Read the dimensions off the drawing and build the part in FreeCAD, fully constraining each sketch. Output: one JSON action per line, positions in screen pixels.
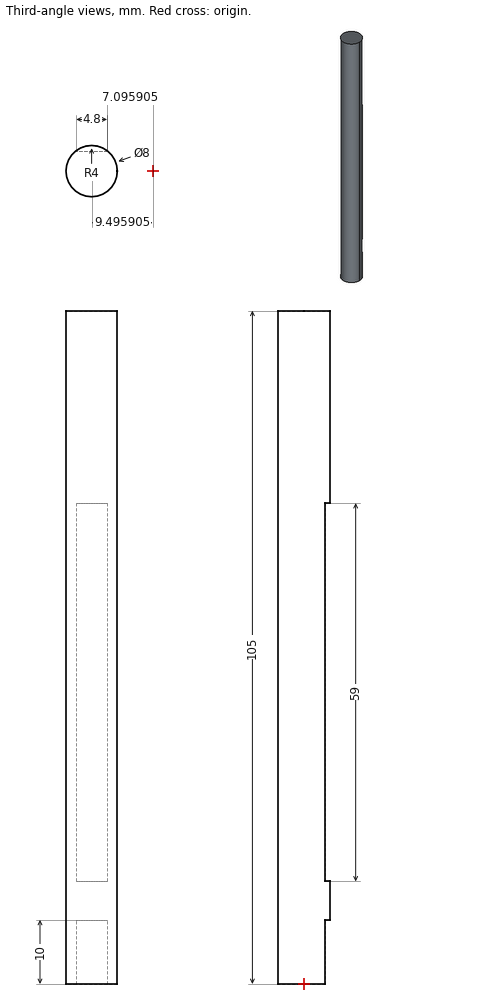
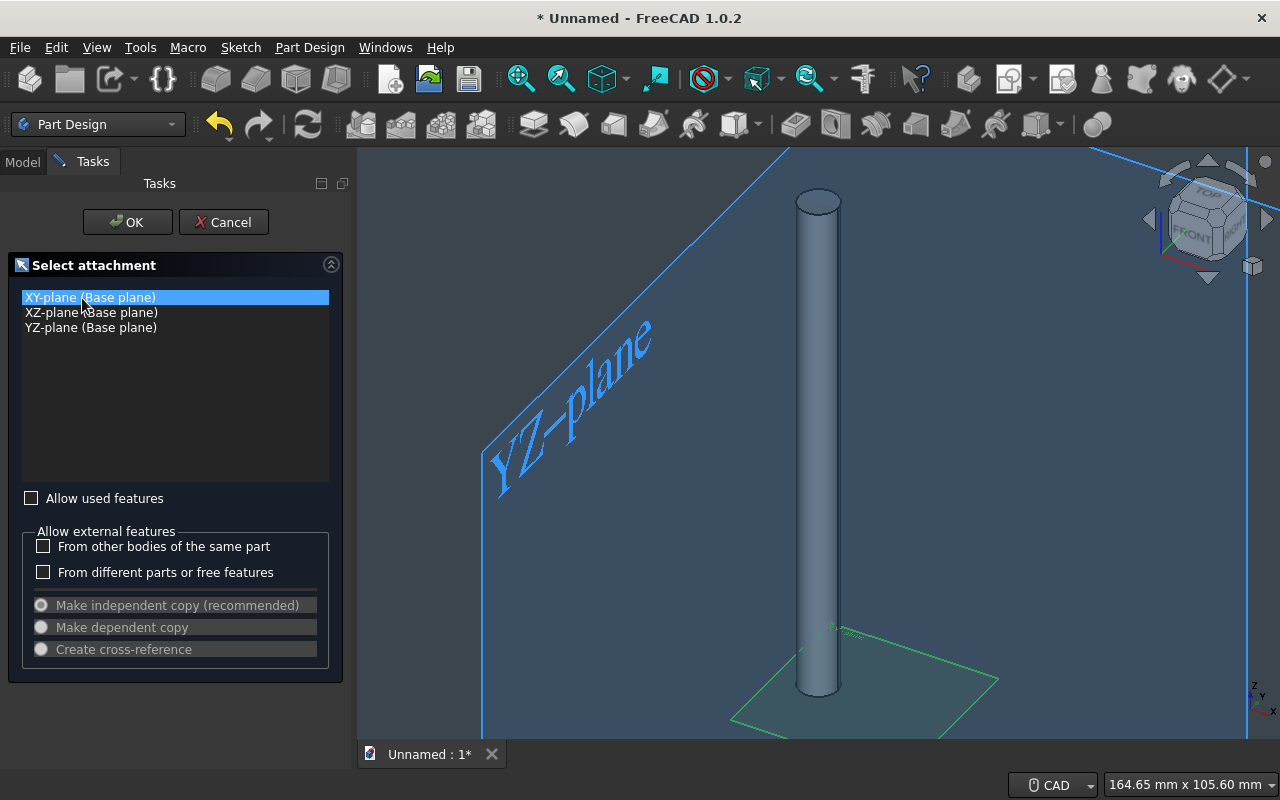
{"action": "left_click", "coordinate": [128, 222]}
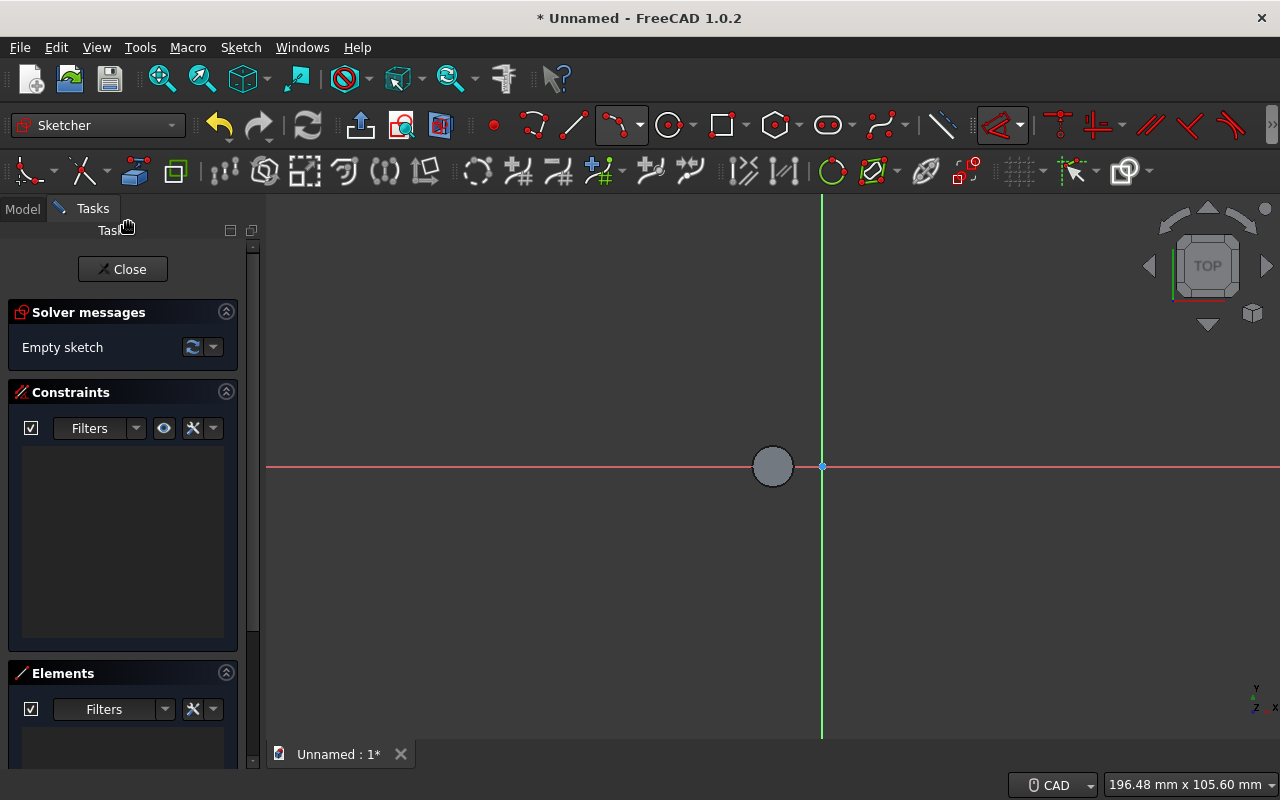
{"action": "key", "text": "q s"}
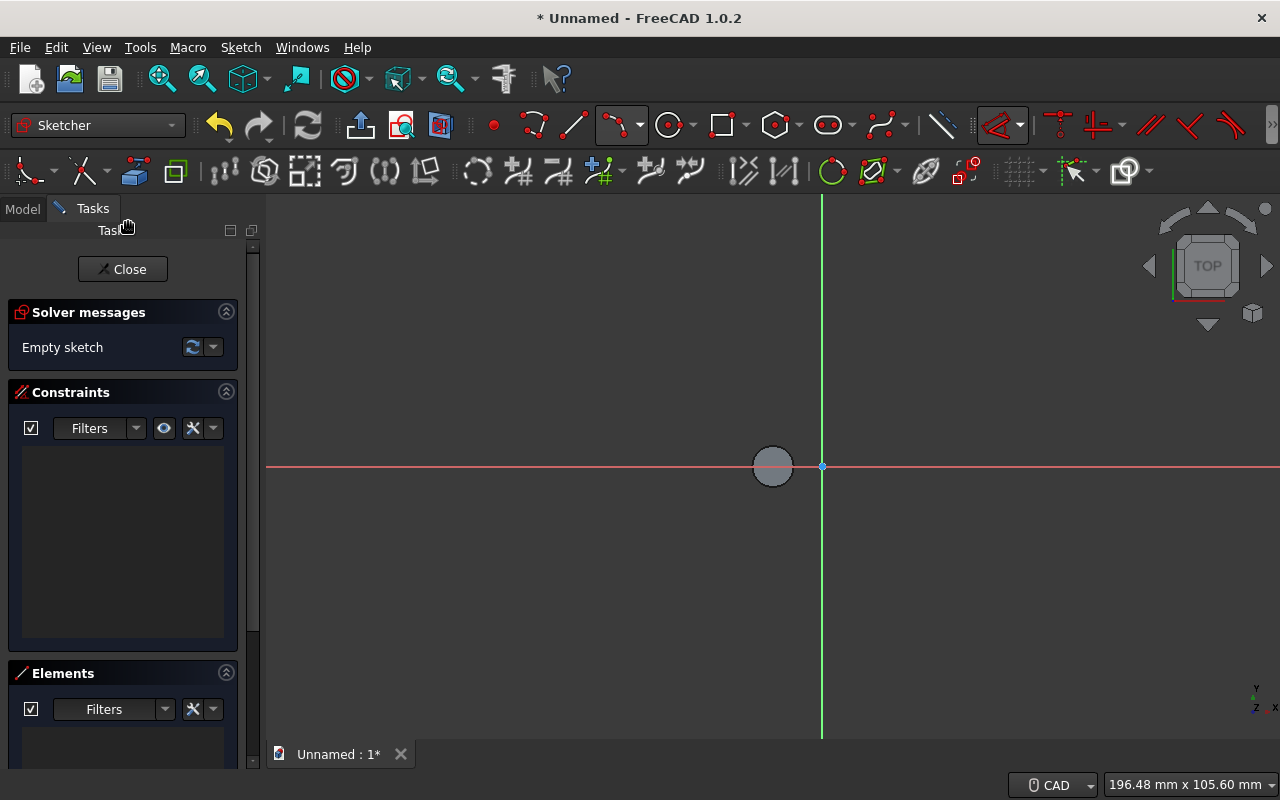
{"action": "scroll", "coordinate": [802, 455], "scroll_direction": "up", "scroll_amount": 11}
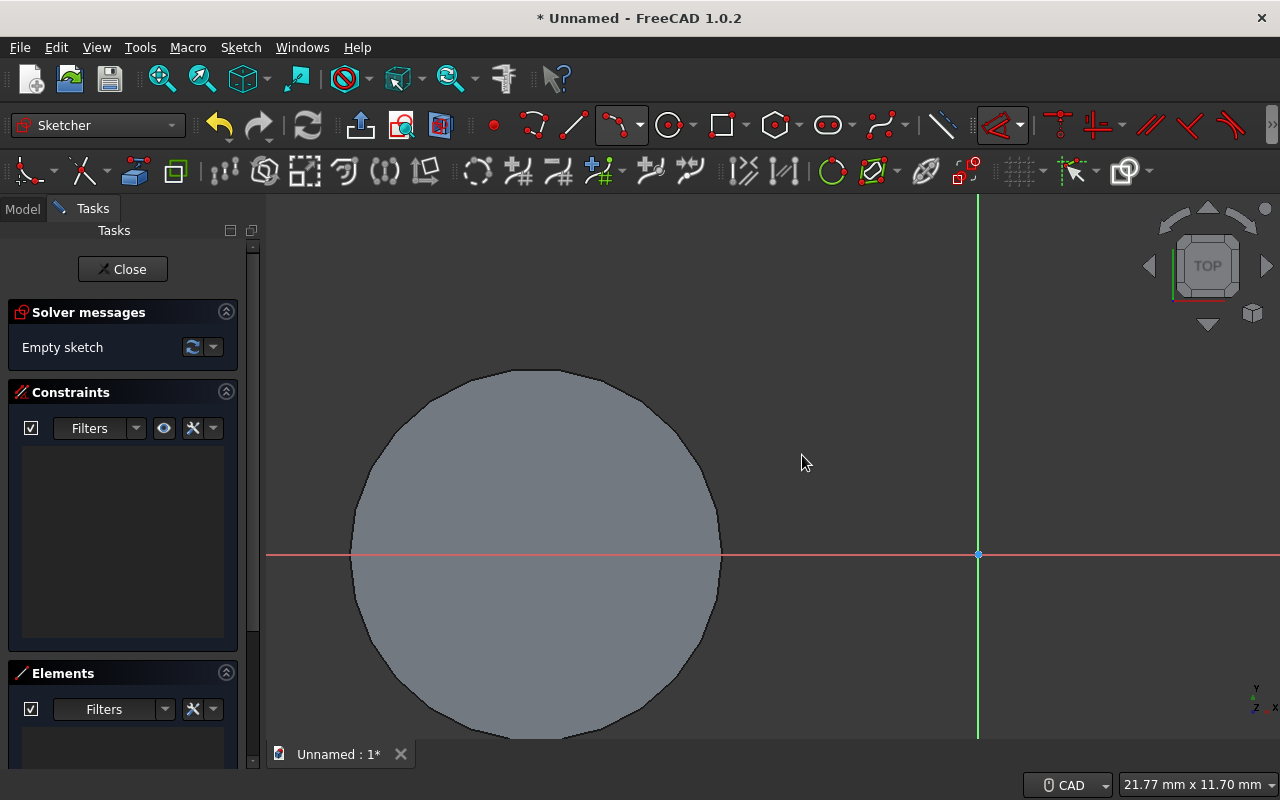
{"action": "key", "text": "g l"}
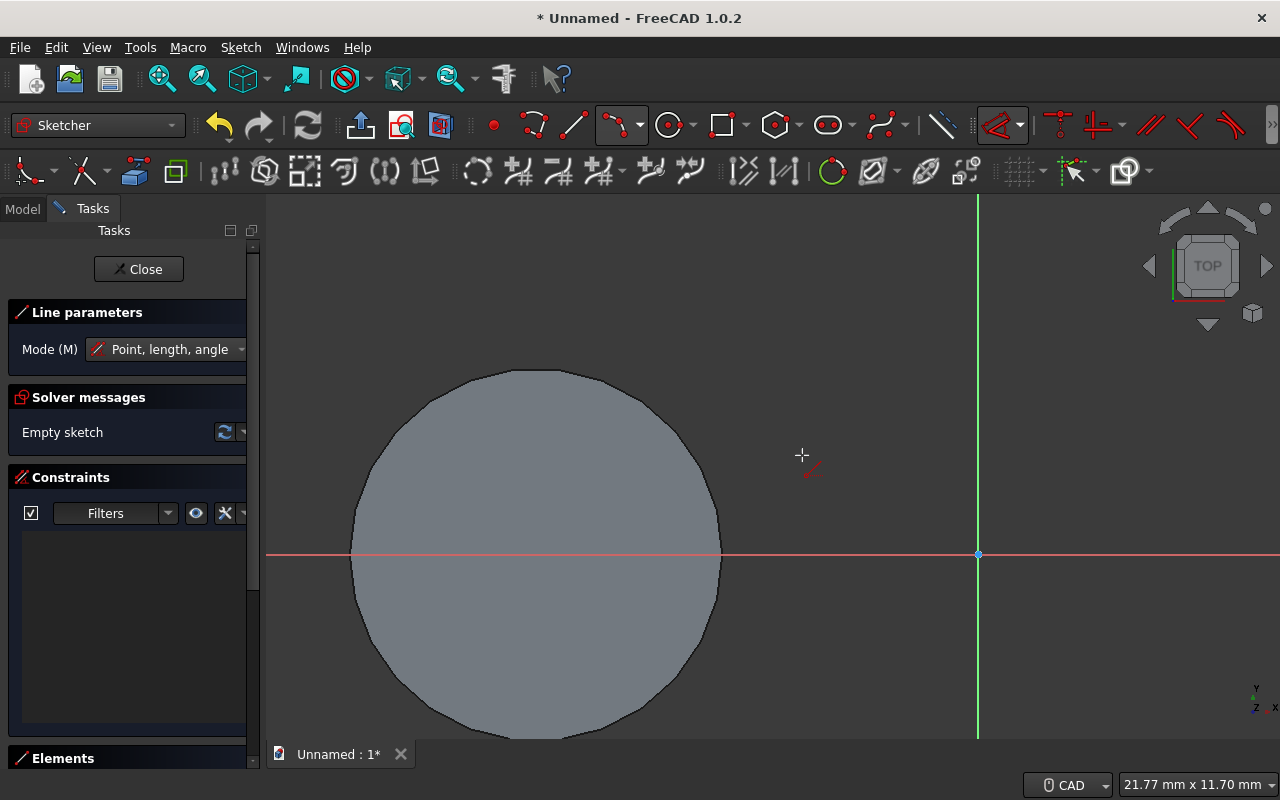
{"action": "left_click", "coordinate": [648, 406]}
{"action": "left_click", "coordinate": [424, 406]}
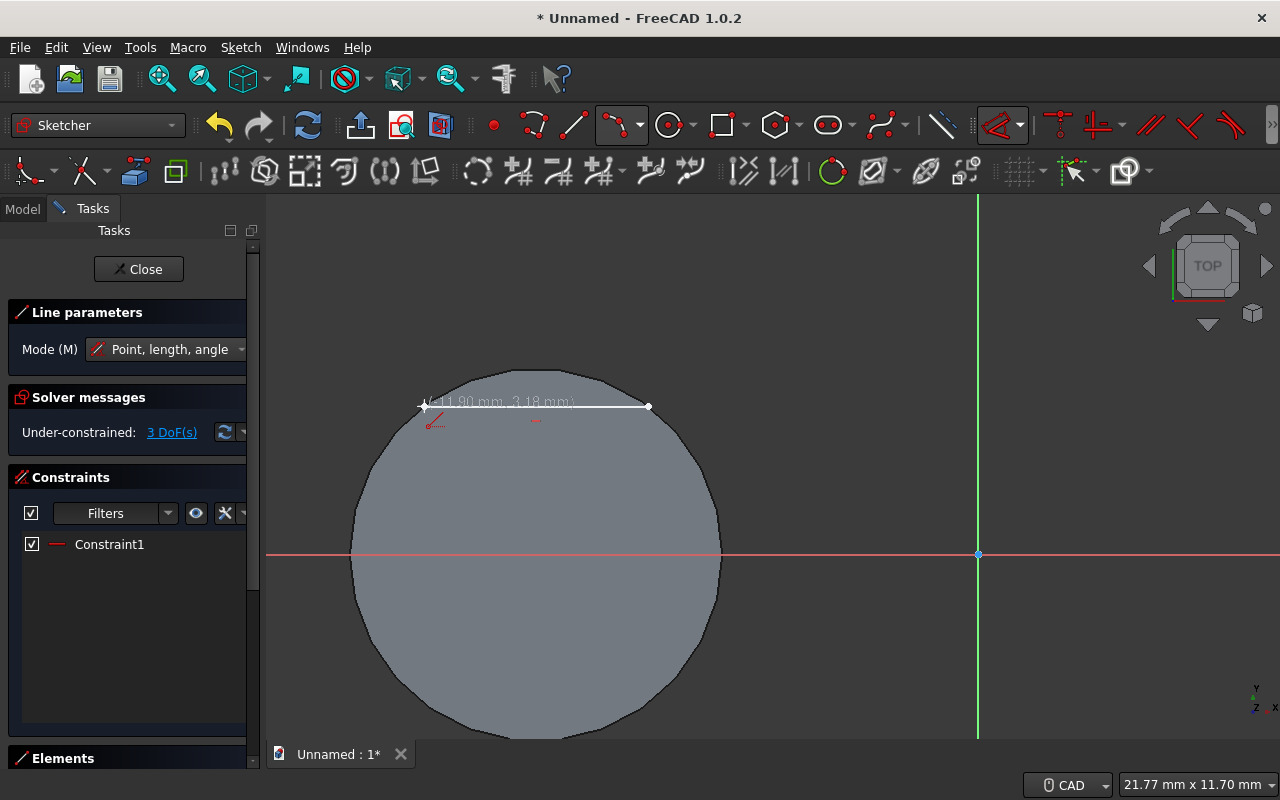
{"action": "key", "text": "g 3 a"}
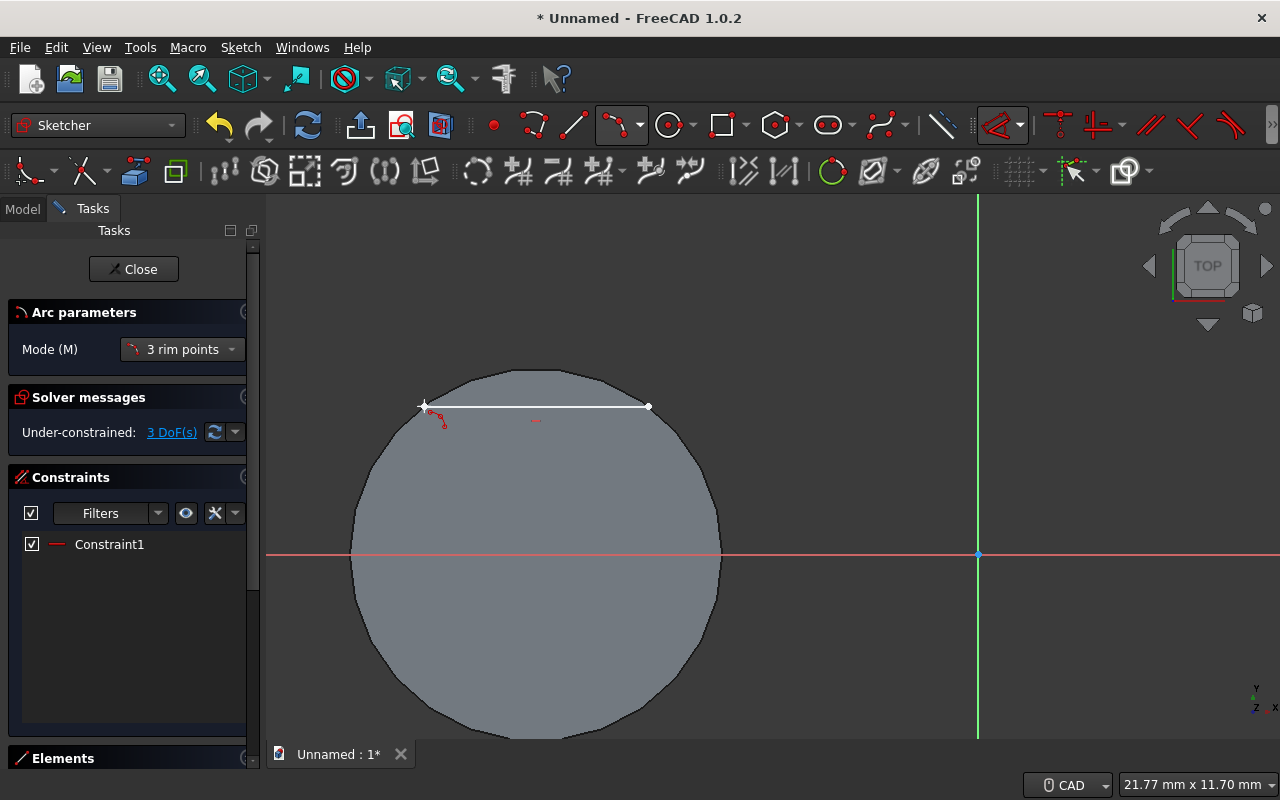
{"action": "left_click", "coordinate": [424, 407]}
{"action": "left_click", "coordinate": [648, 407]}
{"action": "left_click", "coordinate": [536, 369]}
{"action": "key", "text": "Escape"}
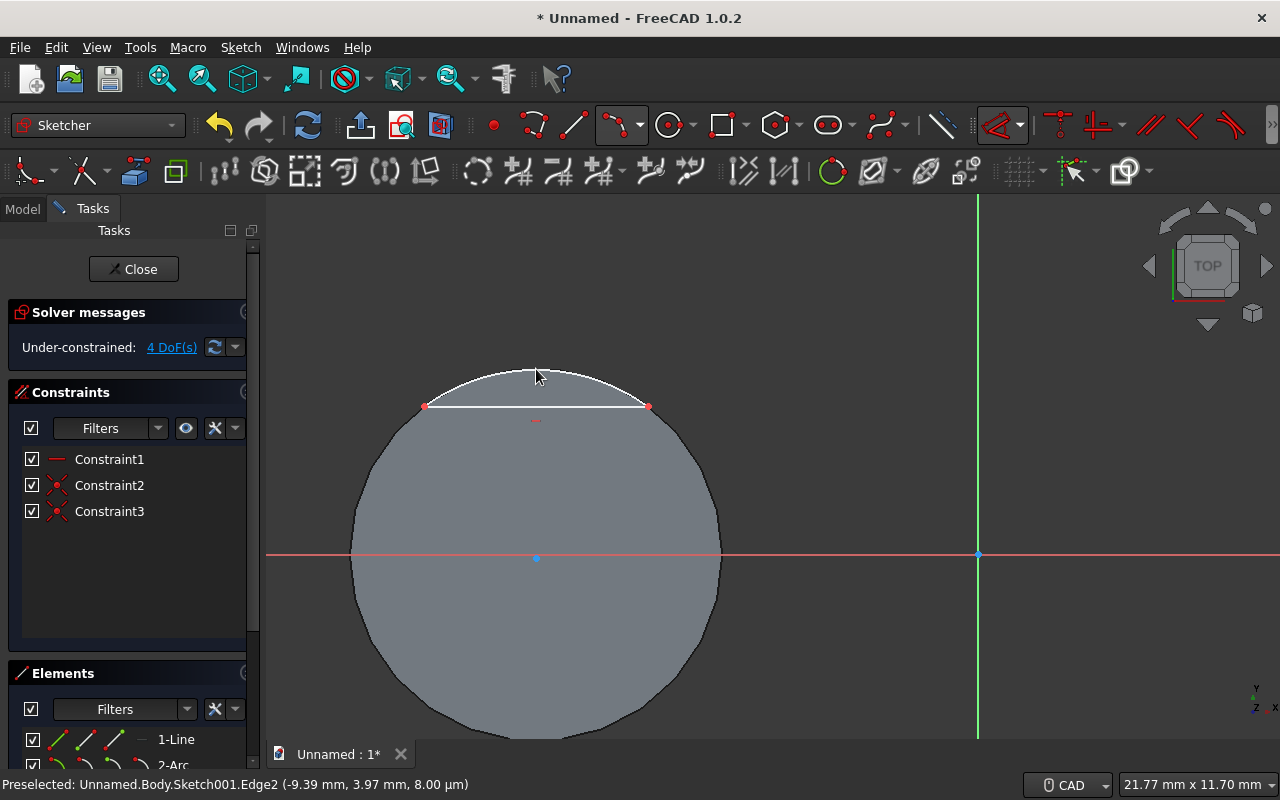
{"action": "left_click", "coordinate": [536, 558]}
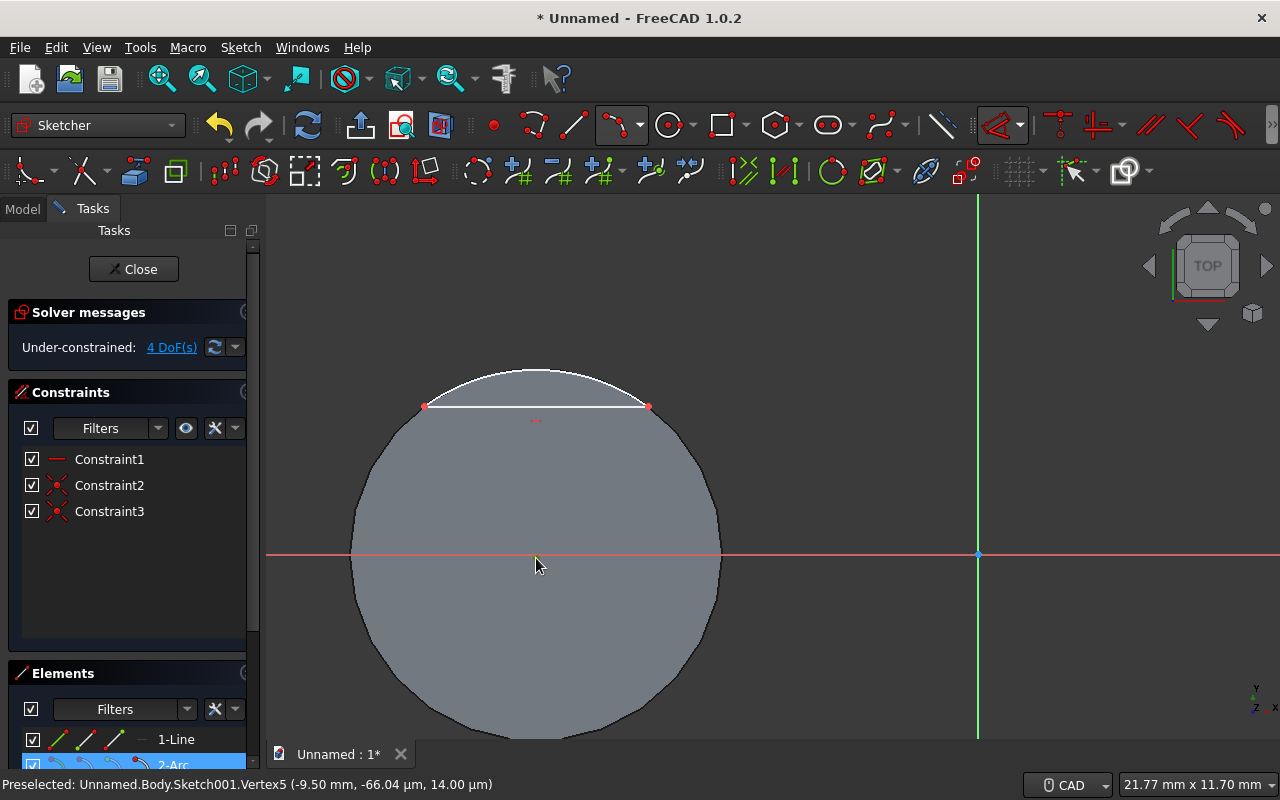
{"action": "left_click", "coordinate": [353, 555]}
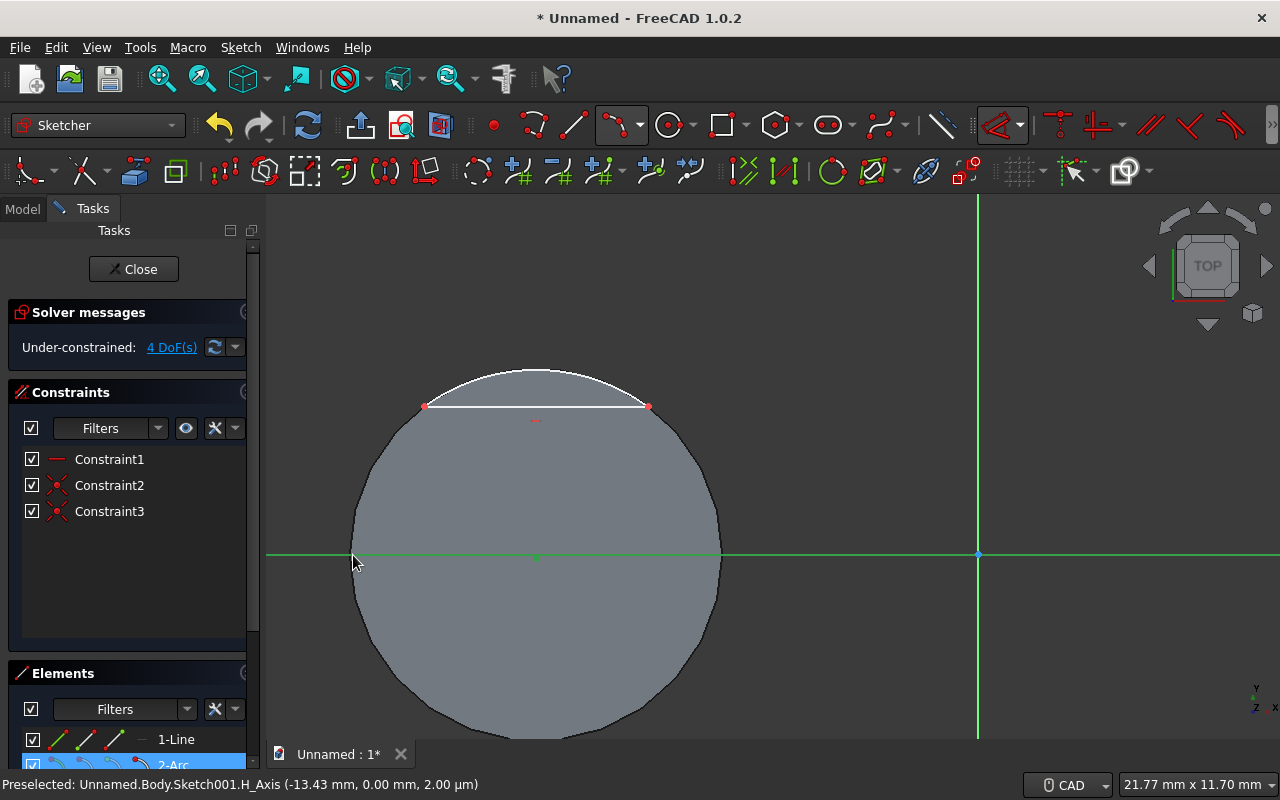
{"action": "key", "text": "c"}